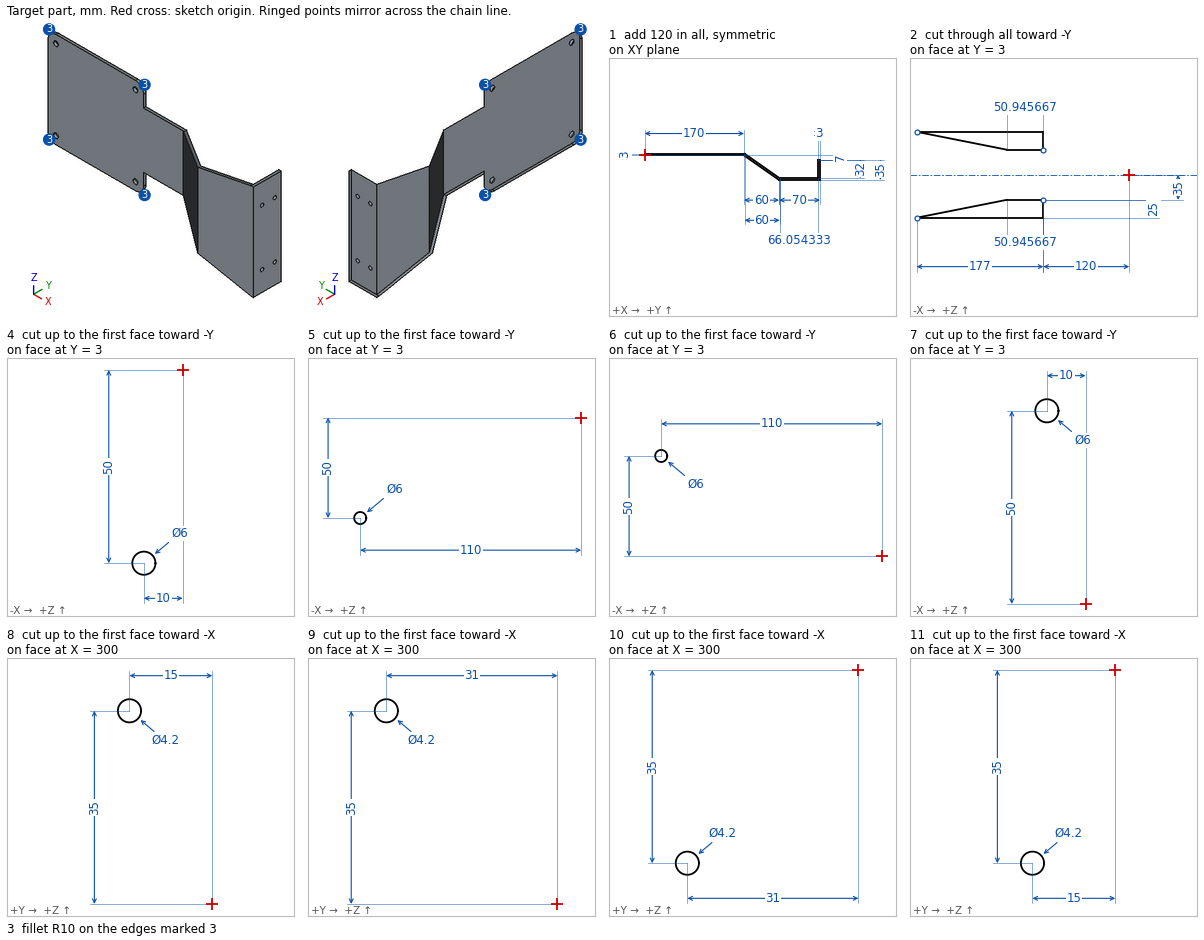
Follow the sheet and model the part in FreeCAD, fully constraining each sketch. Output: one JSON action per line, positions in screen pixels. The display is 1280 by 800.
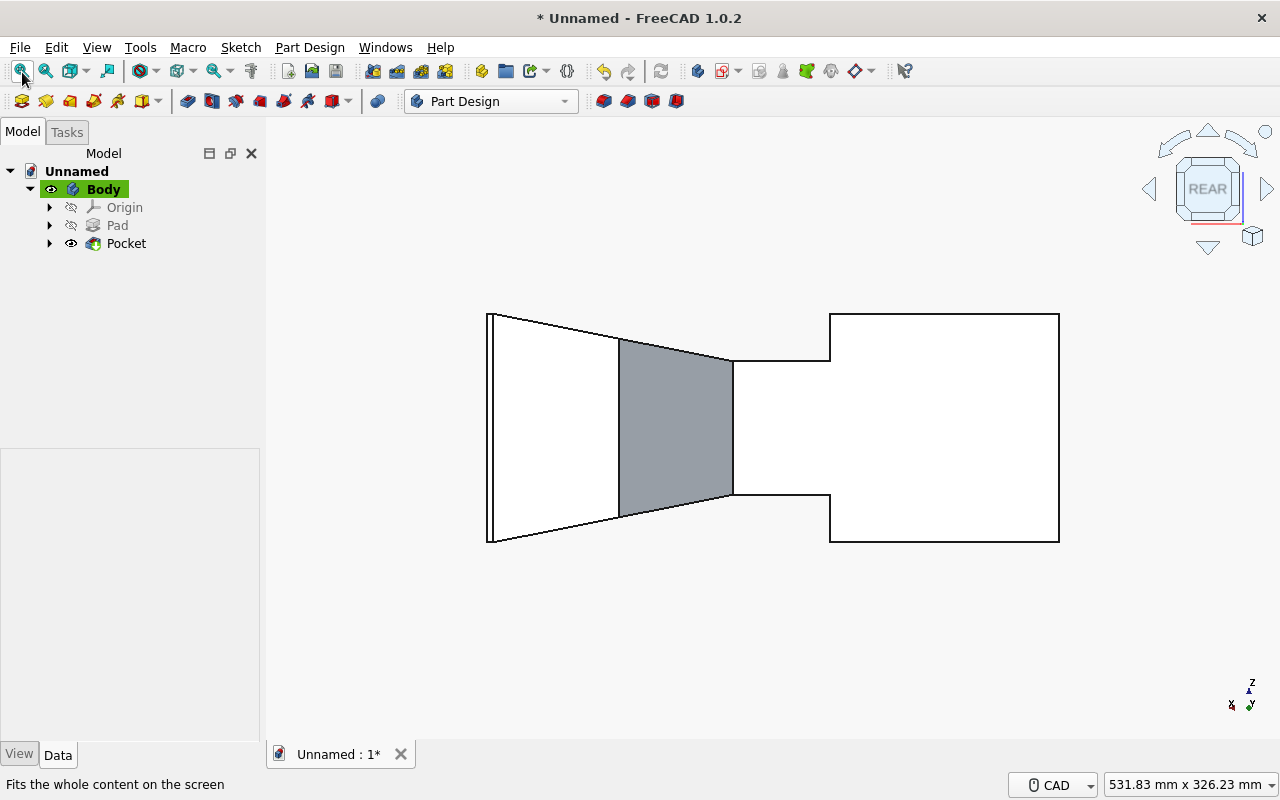
{"action": "key", "text": "0"}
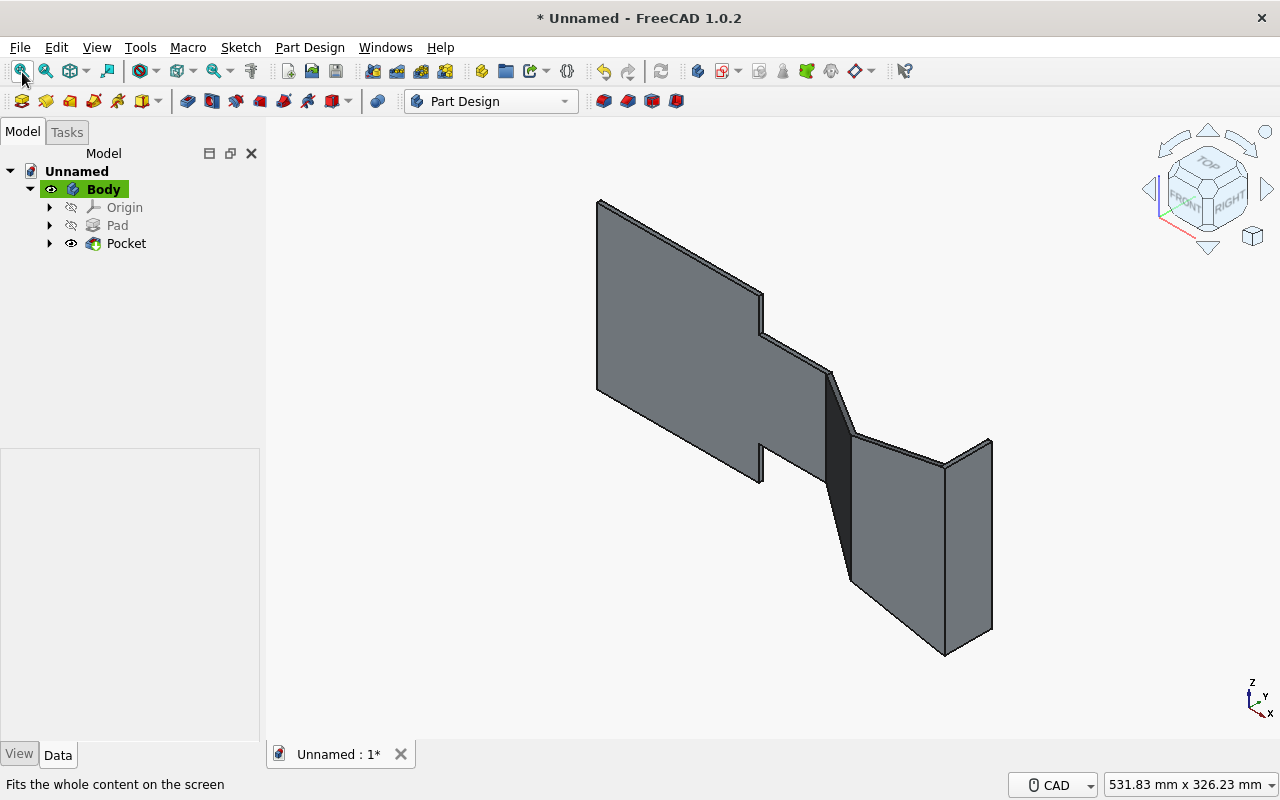
{"action": "scroll", "coordinate": [599, 387], "scroll_direction": "up", "scroll_amount": 10}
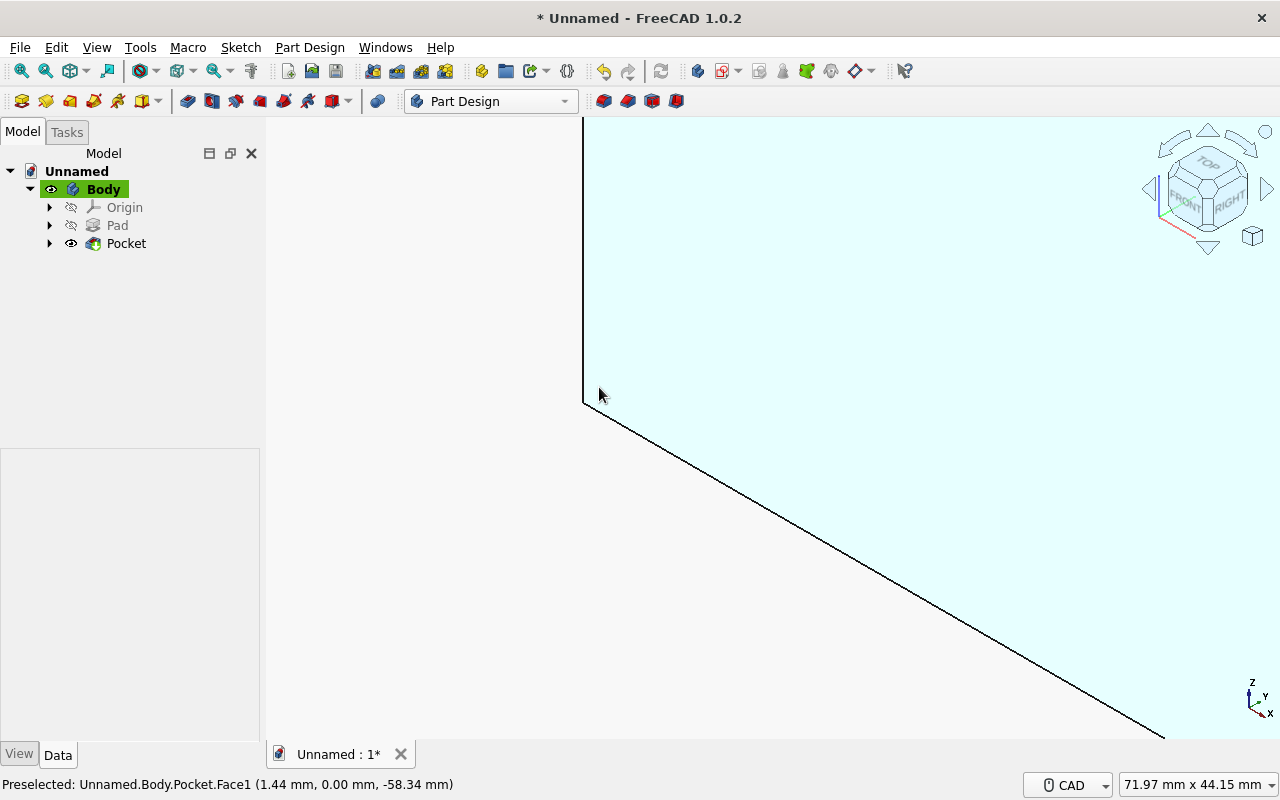
{"action": "left_click", "coordinate": [22, 72]}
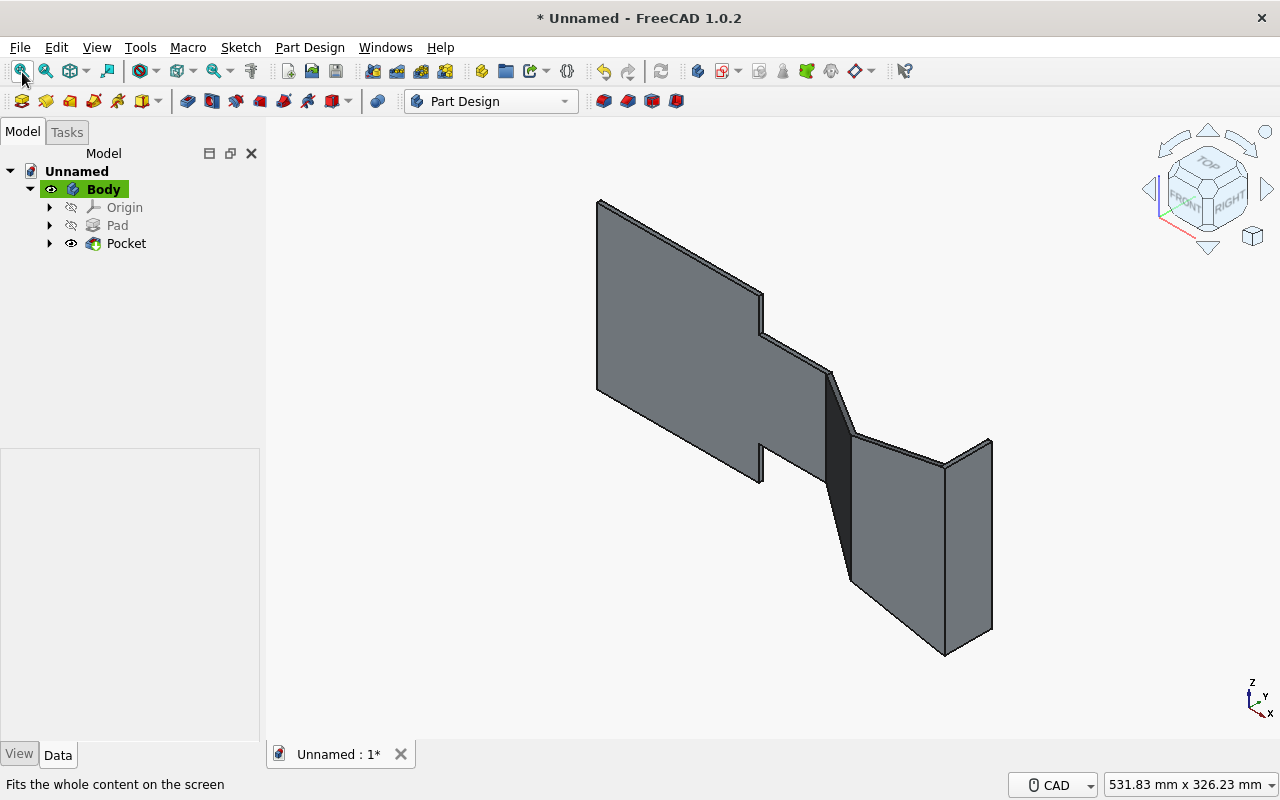
{"action": "key", "text": "2"}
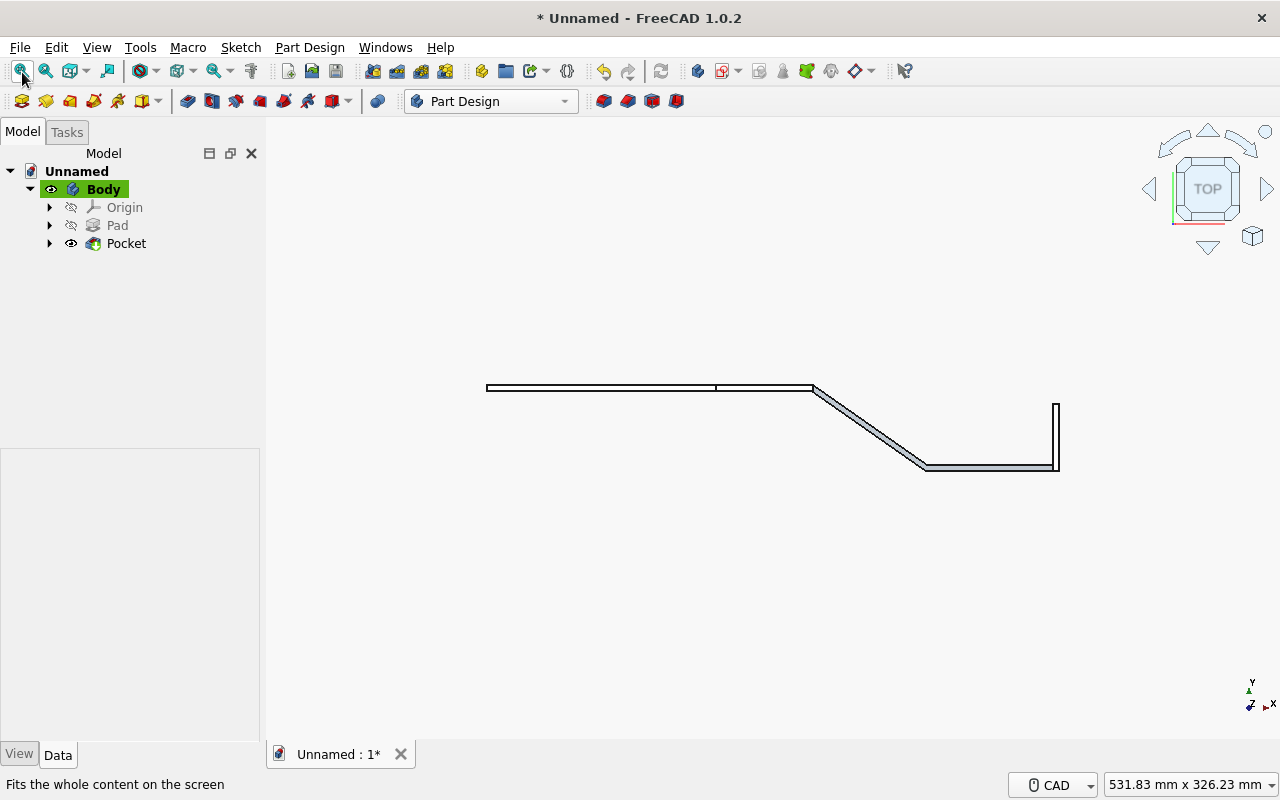
{"action": "scroll", "coordinate": [487, 387], "scroll_direction": "up", "scroll_amount": 10}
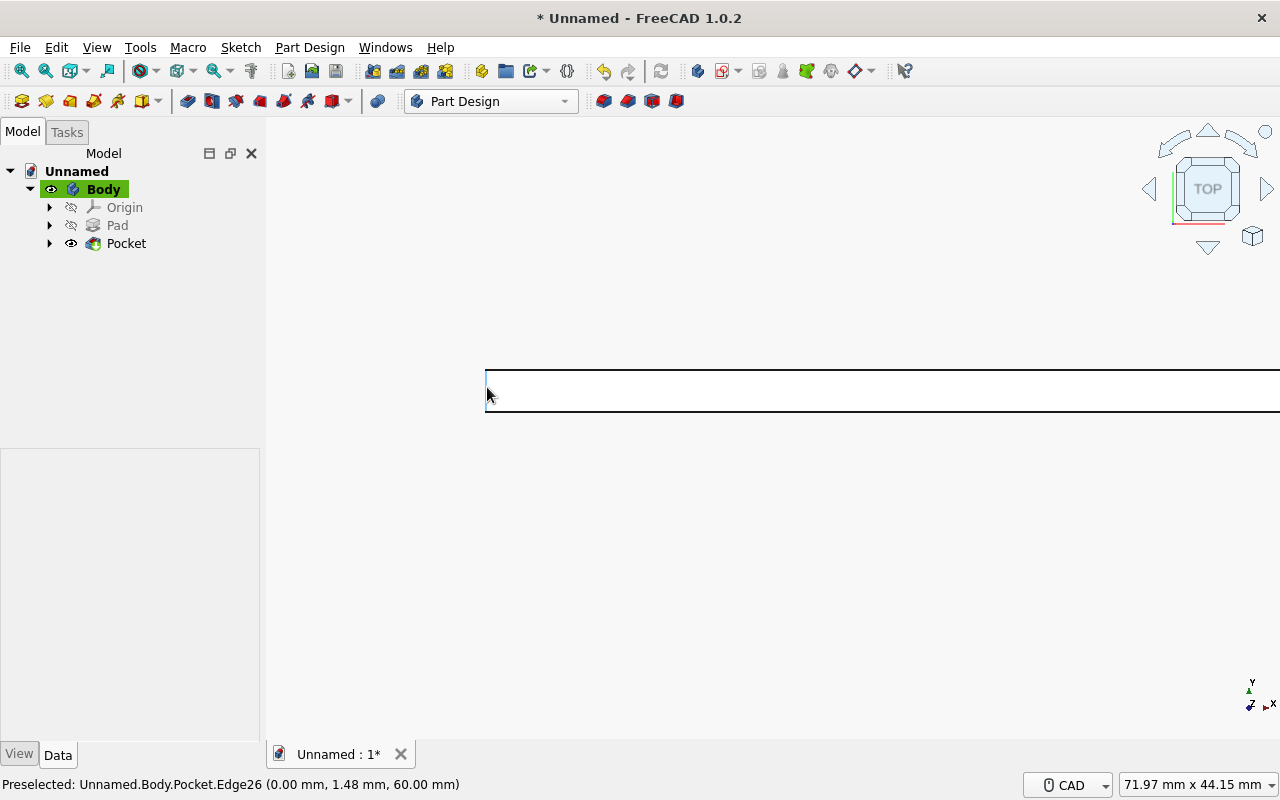
{"action": "left_click", "coordinate": [486, 390]}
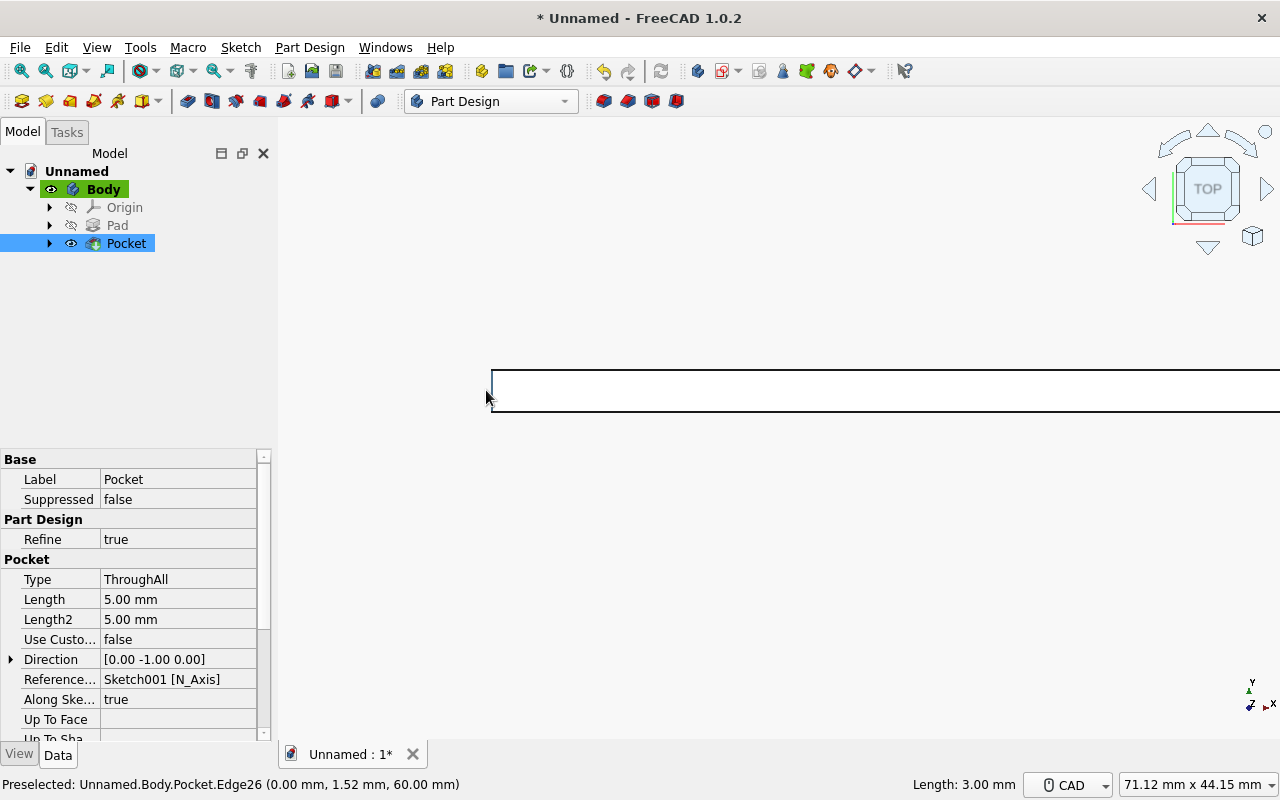
{"action": "left_click", "coordinate": [22, 72]}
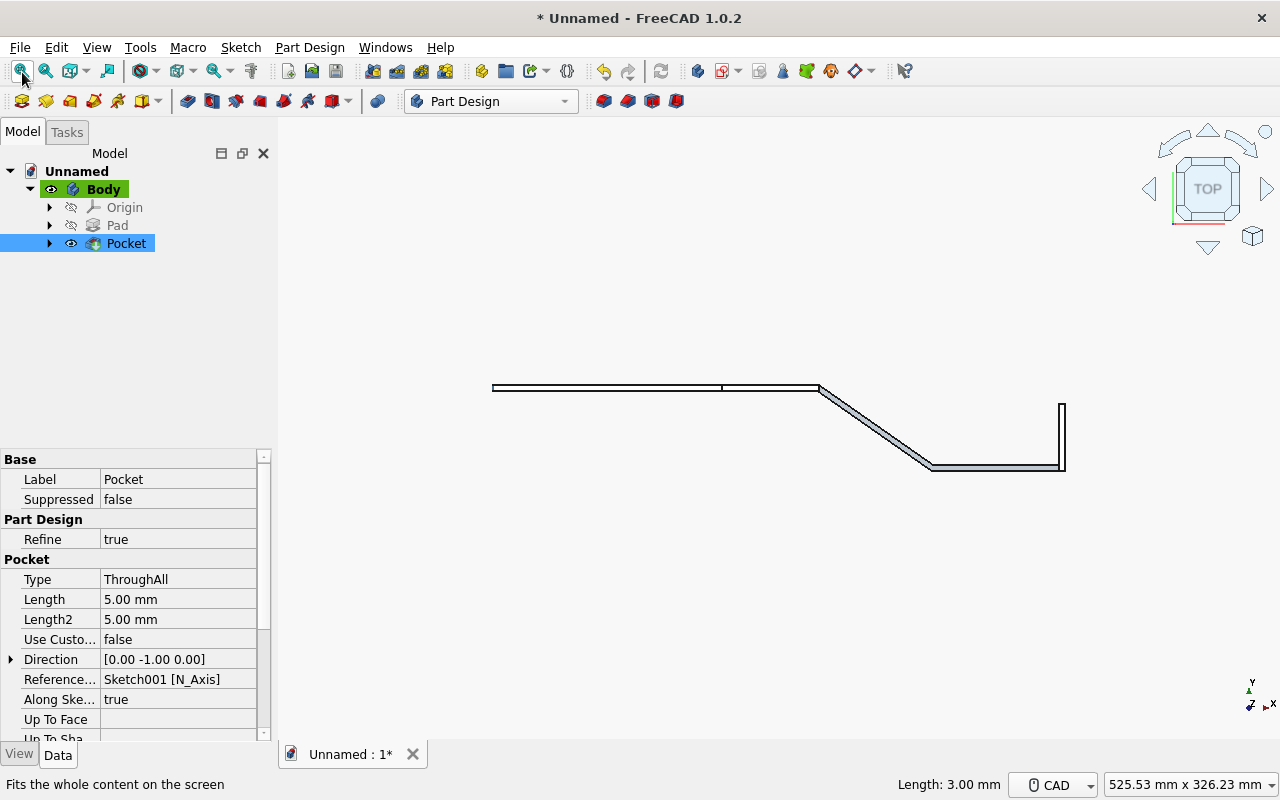
{"action": "key", "text": "1"}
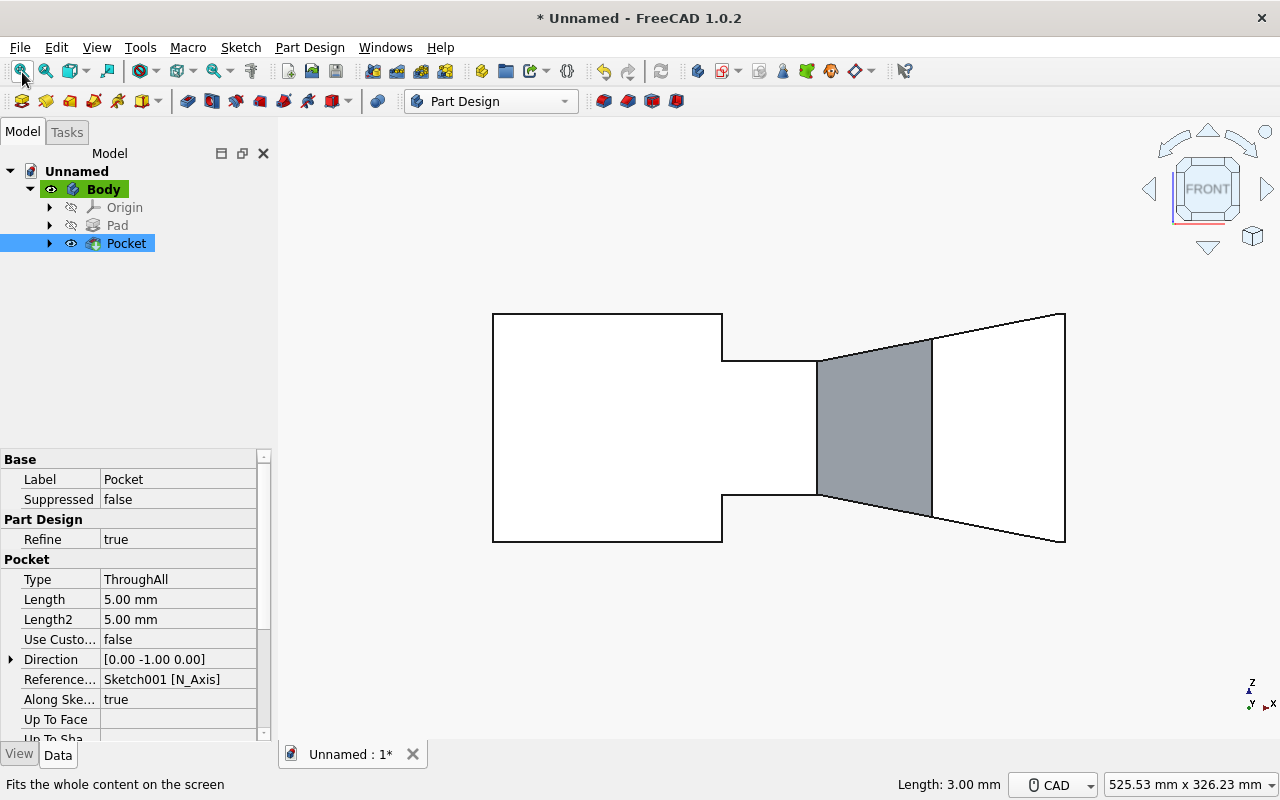
{"action": "scroll", "coordinate": [493, 541], "scroll_direction": "up", "scroll_amount": 10}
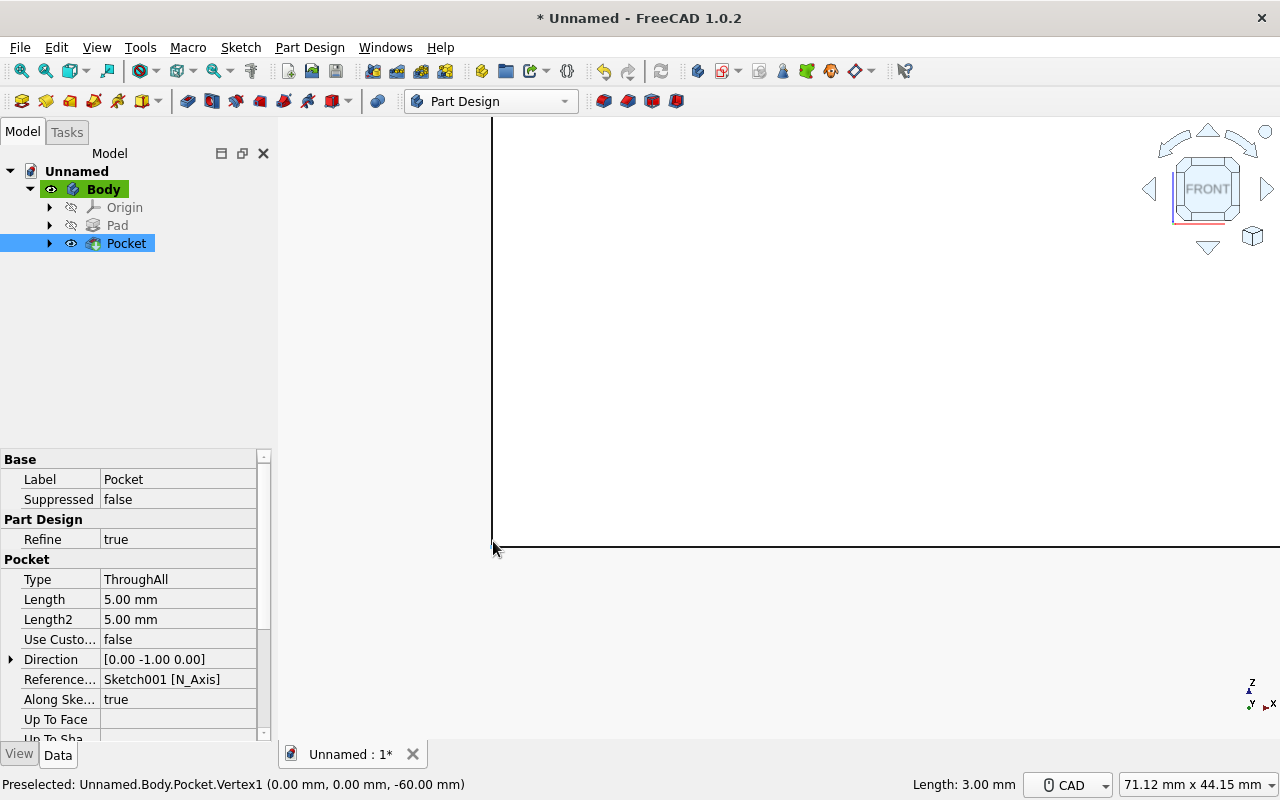
{"action": "left_click", "coordinate": [22, 72]}